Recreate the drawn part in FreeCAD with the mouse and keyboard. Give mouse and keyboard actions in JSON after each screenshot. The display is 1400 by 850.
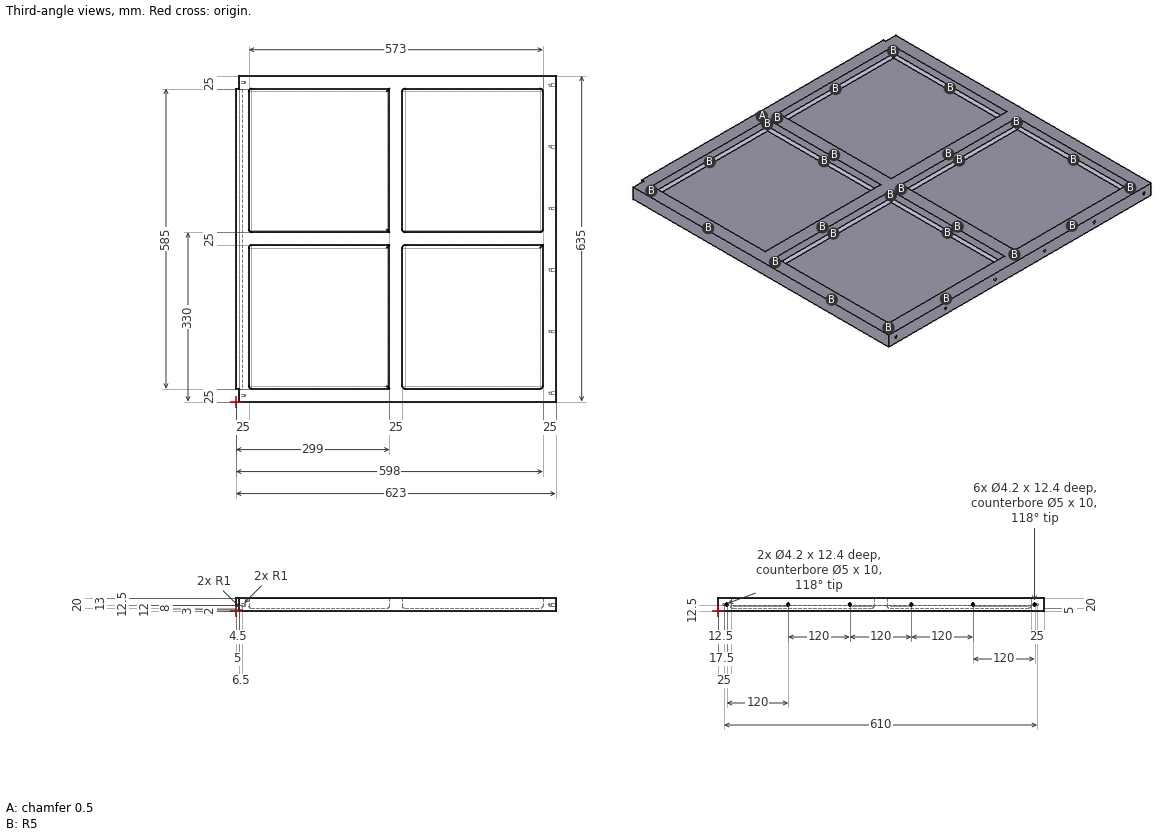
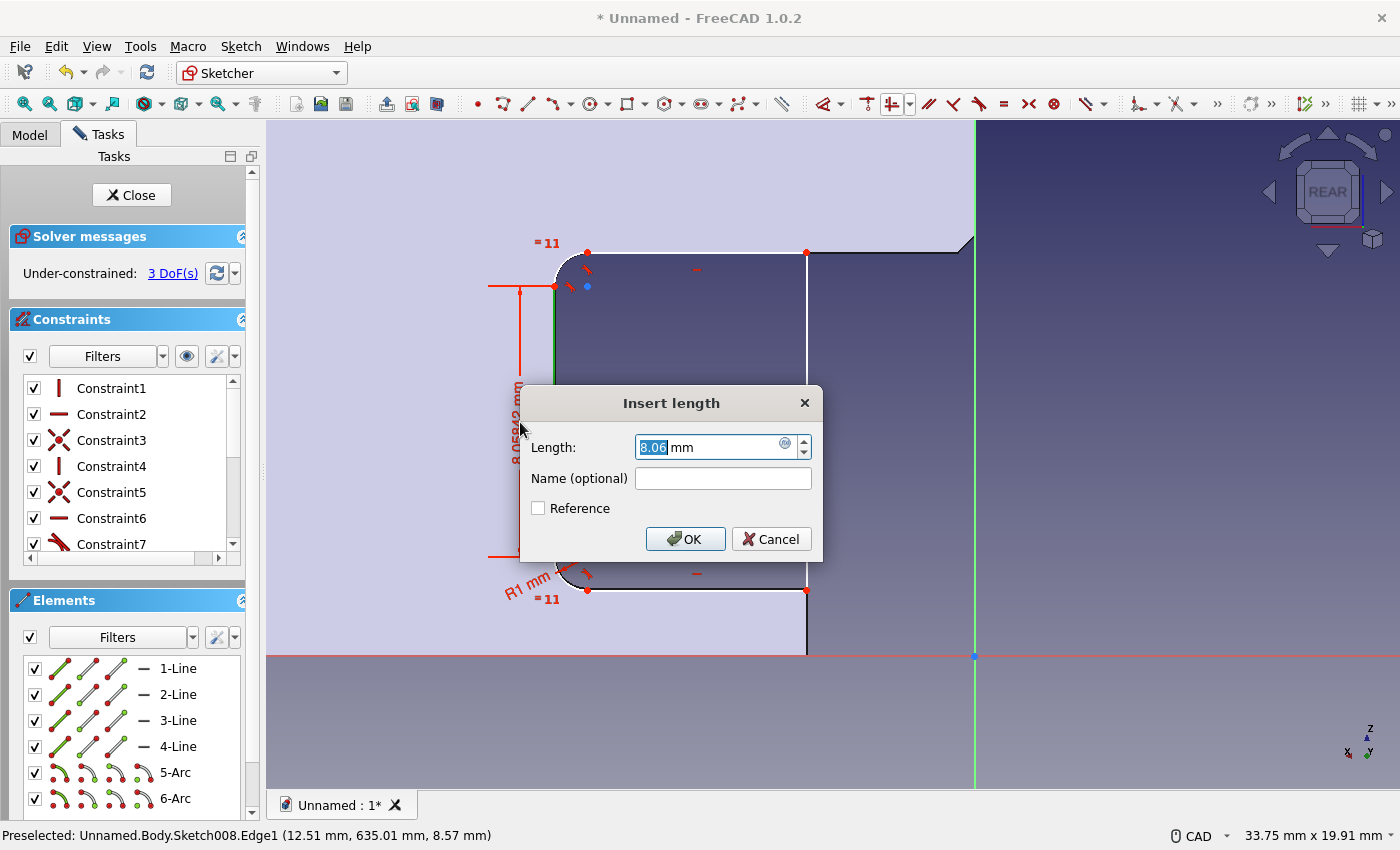
{"action": "type", "text": "8"}
{"action": "key", "text": "Return"}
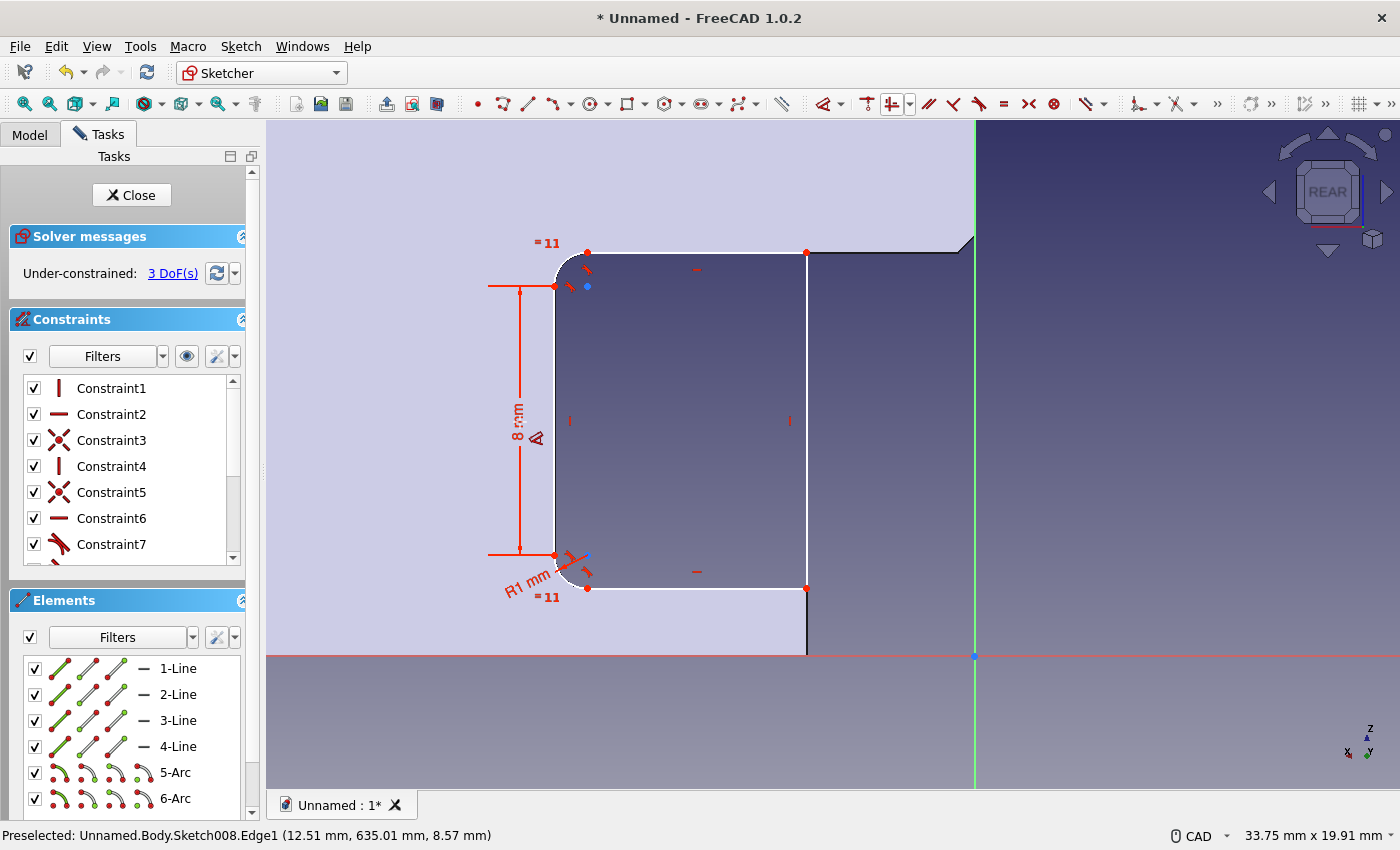
{"action": "left_click", "coordinate": [554, 555]}
{"action": "left_click", "coordinate": [520, 629]}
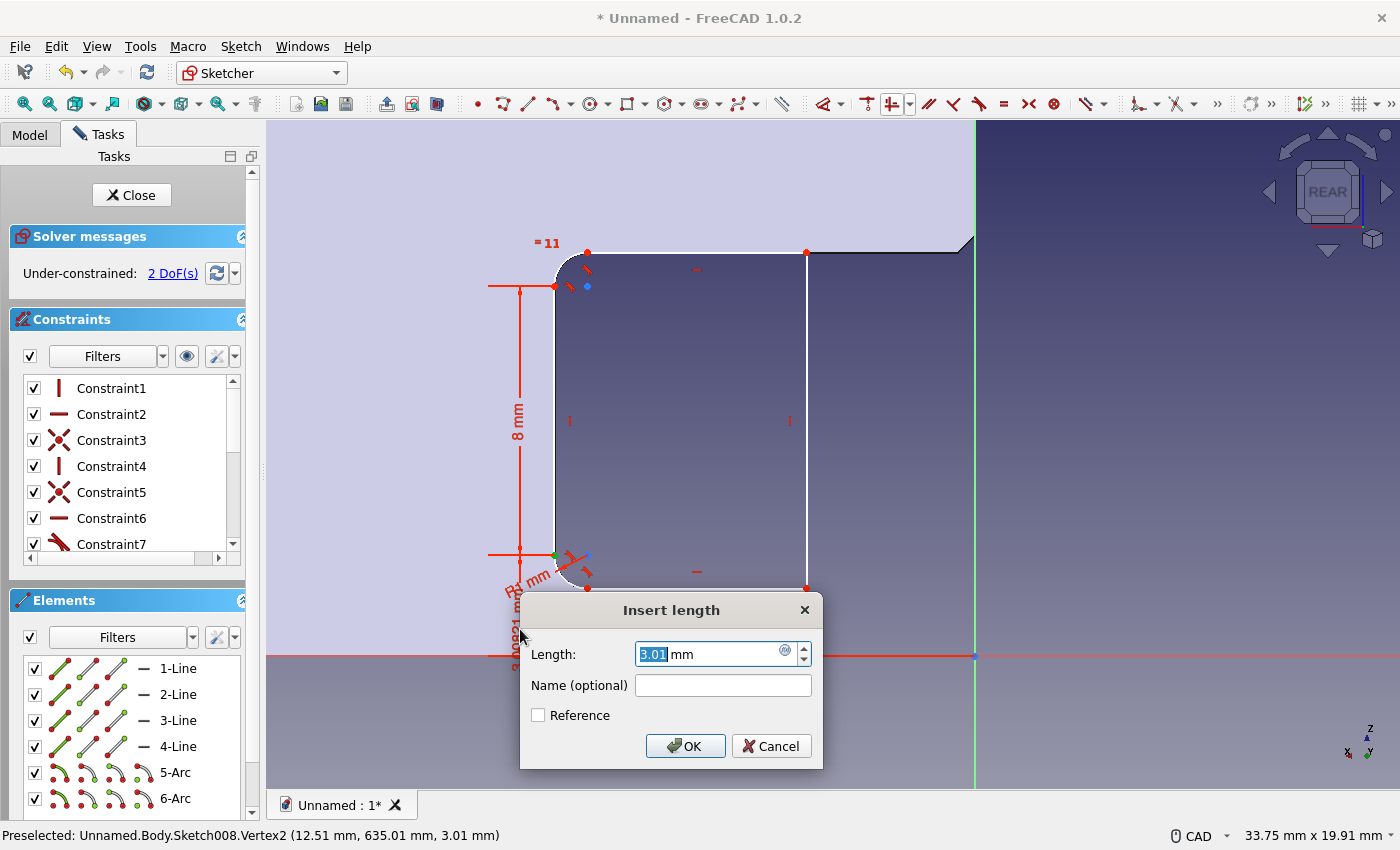
{"action": "type", "text": "3"}
{"action": "key", "text": "Return"}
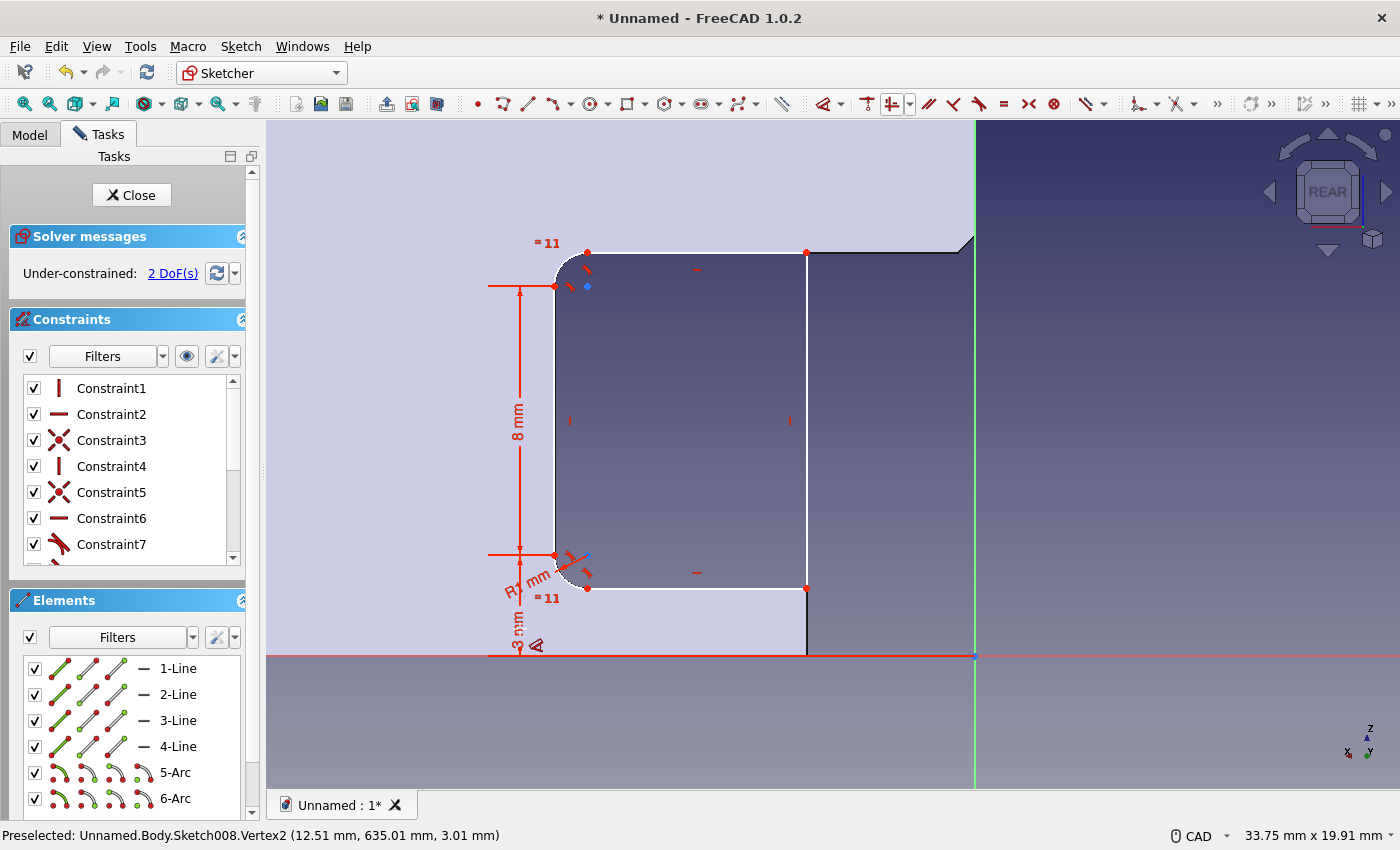
{"action": "left_click", "coordinate": [807, 589]}
{"action": "left_click", "coordinate": [891, 690]}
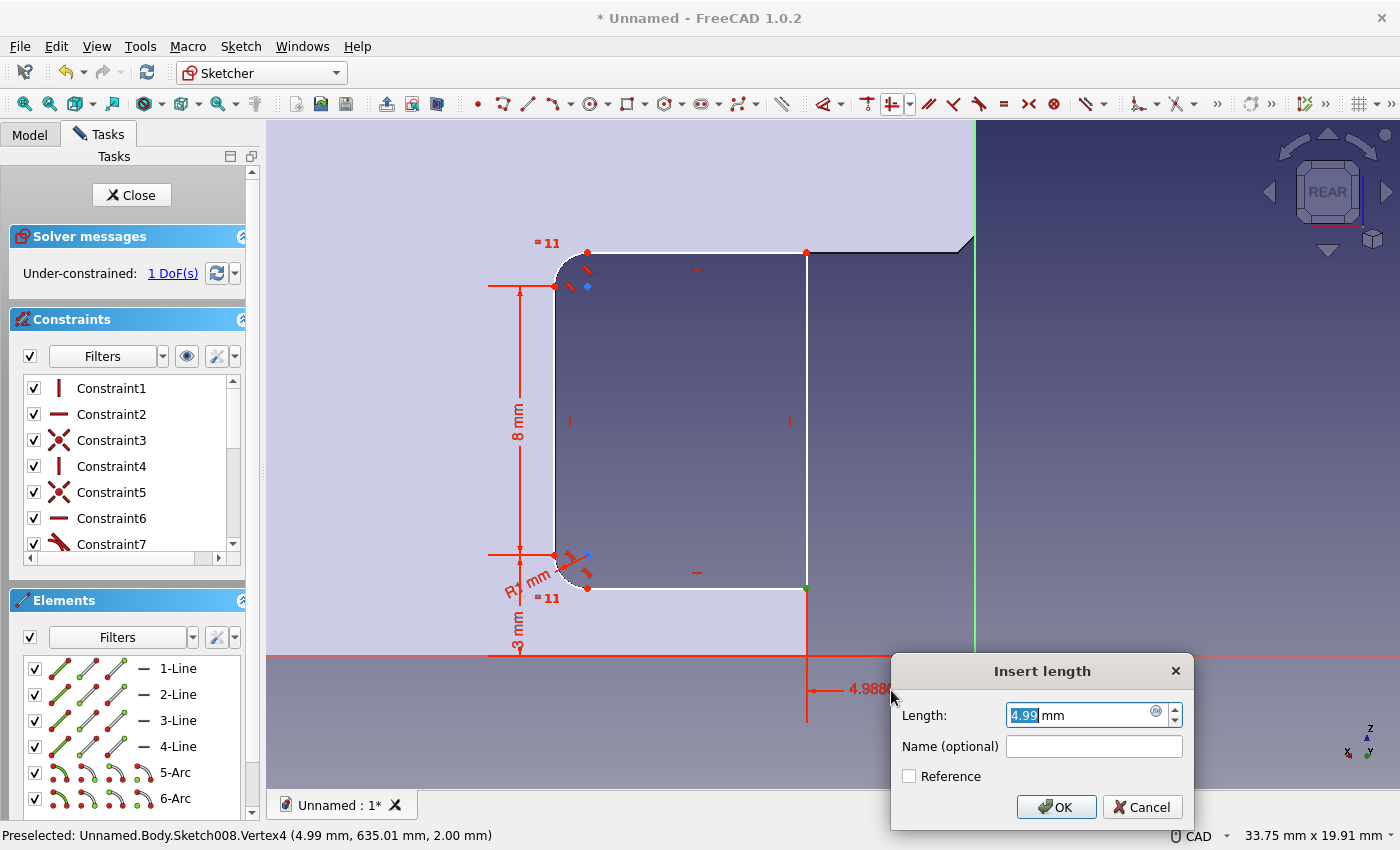
{"action": "type", "text": "5"}
{"action": "key", "text": "Return"}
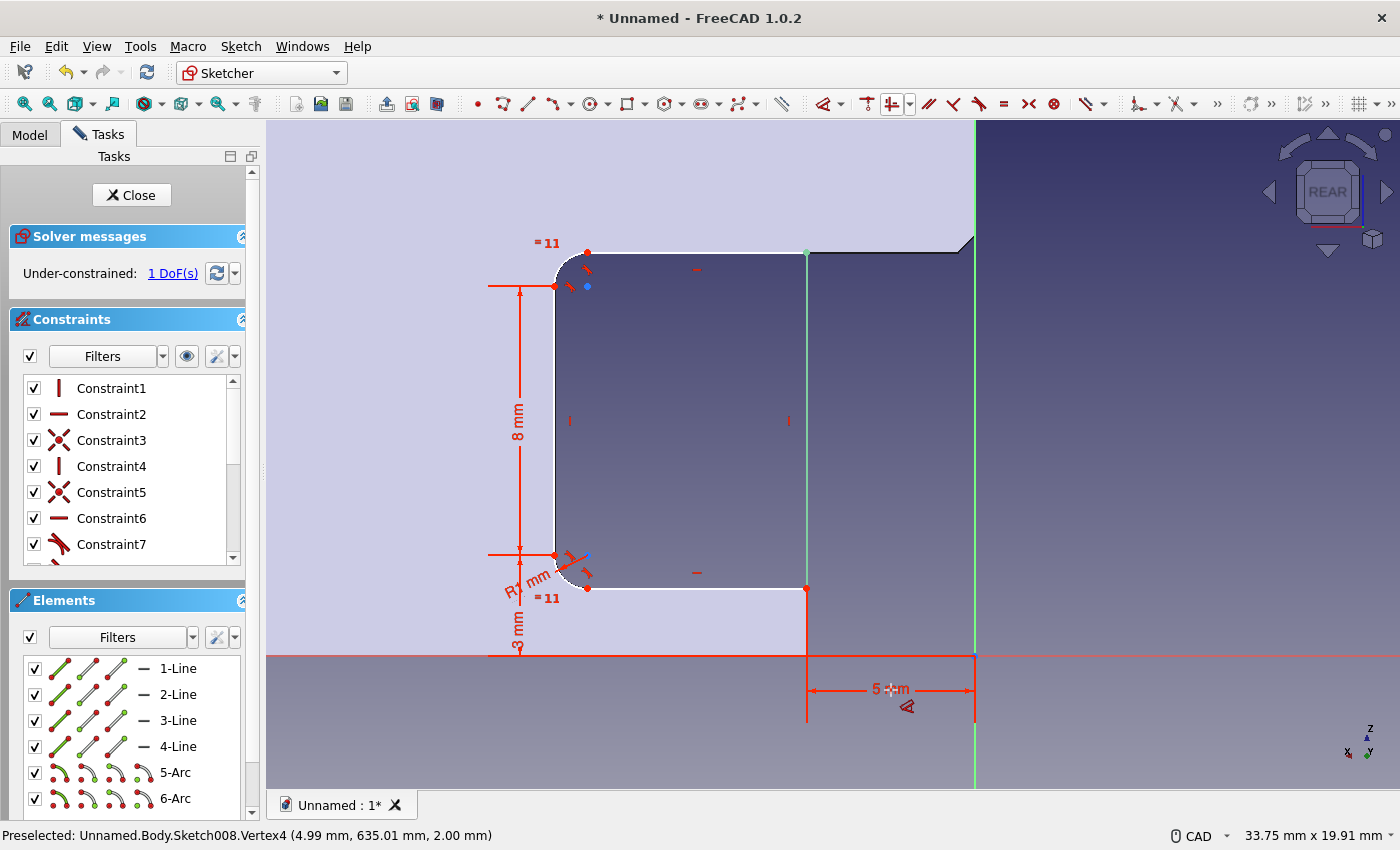
{"action": "left_click", "coordinate": [653, 589]}
{"action": "left_click", "coordinate": [697, 623]}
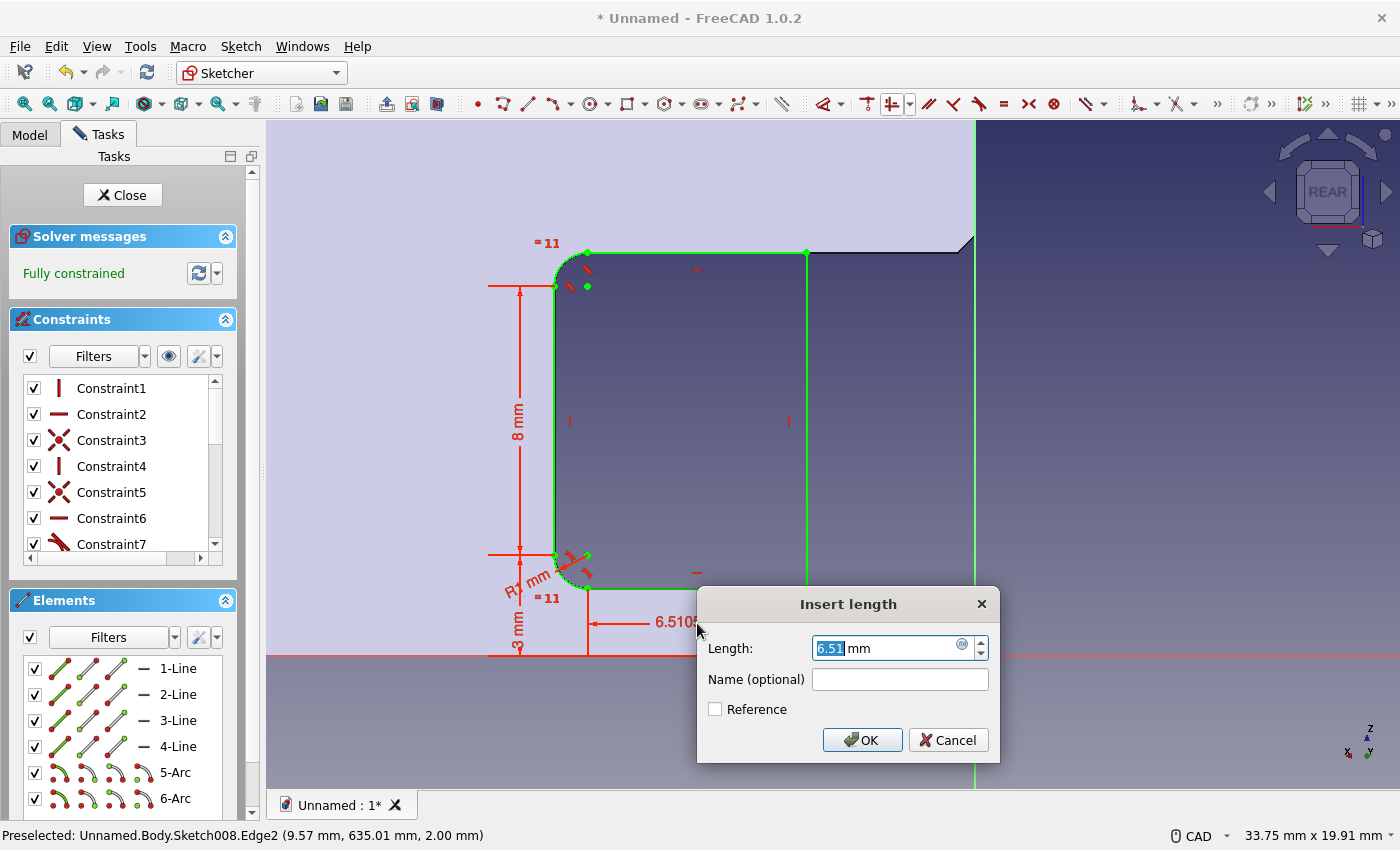
{"action": "type", "text": "6.5"}
{"action": "key", "text": "Return"}
{"action": "key", "text": "Escape"}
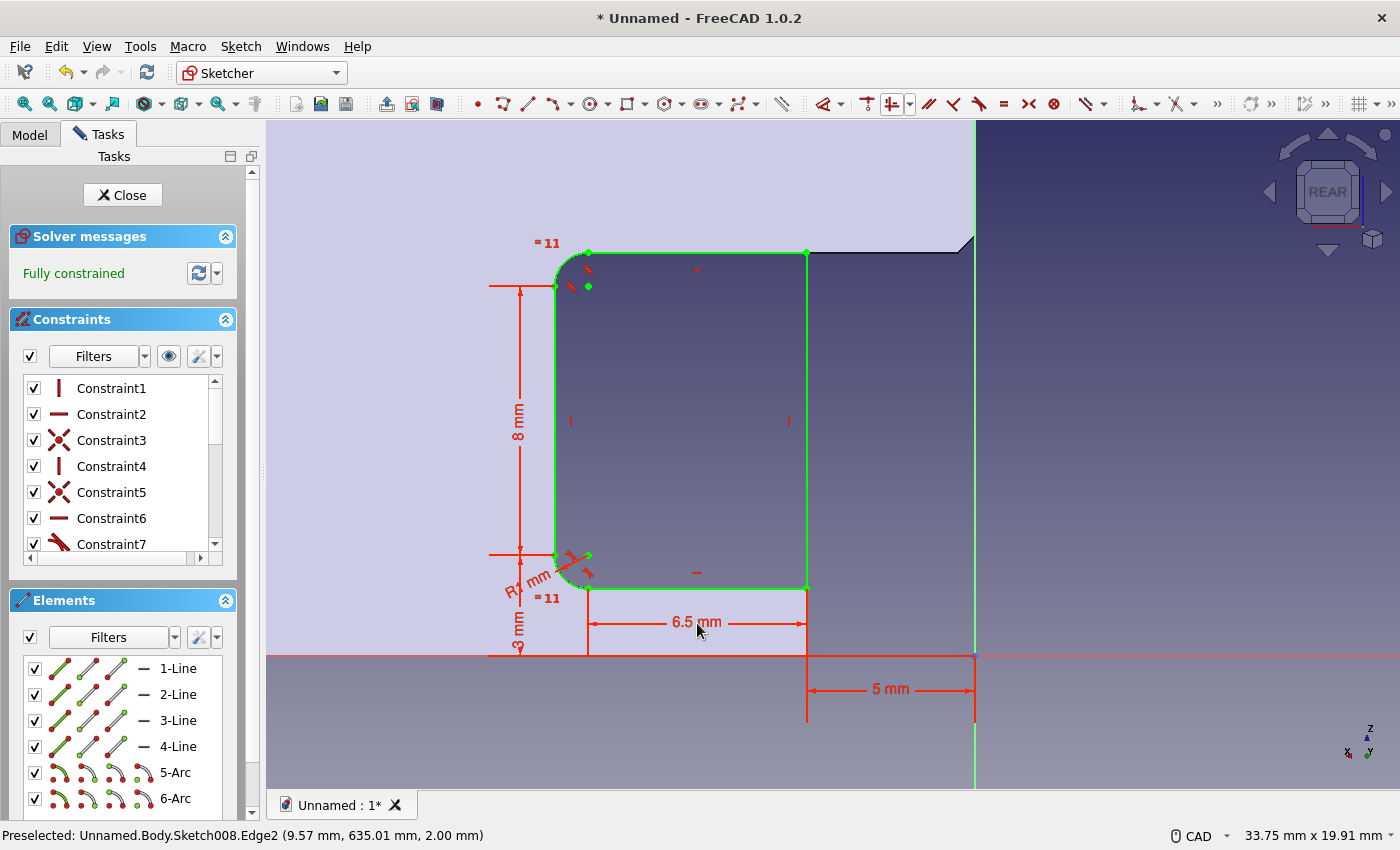
{"action": "left_click", "coordinate": [123, 195]}